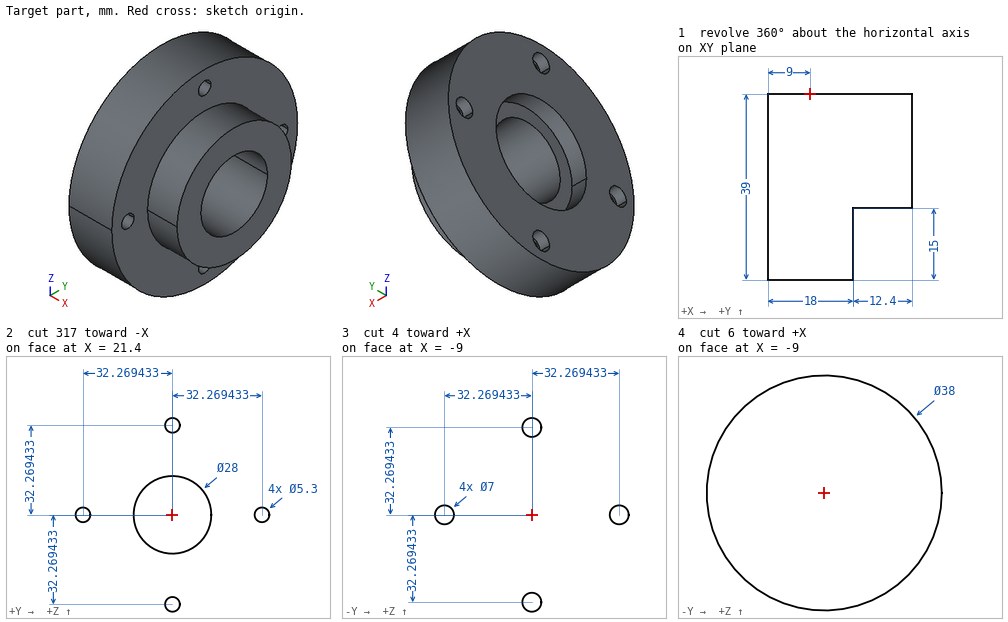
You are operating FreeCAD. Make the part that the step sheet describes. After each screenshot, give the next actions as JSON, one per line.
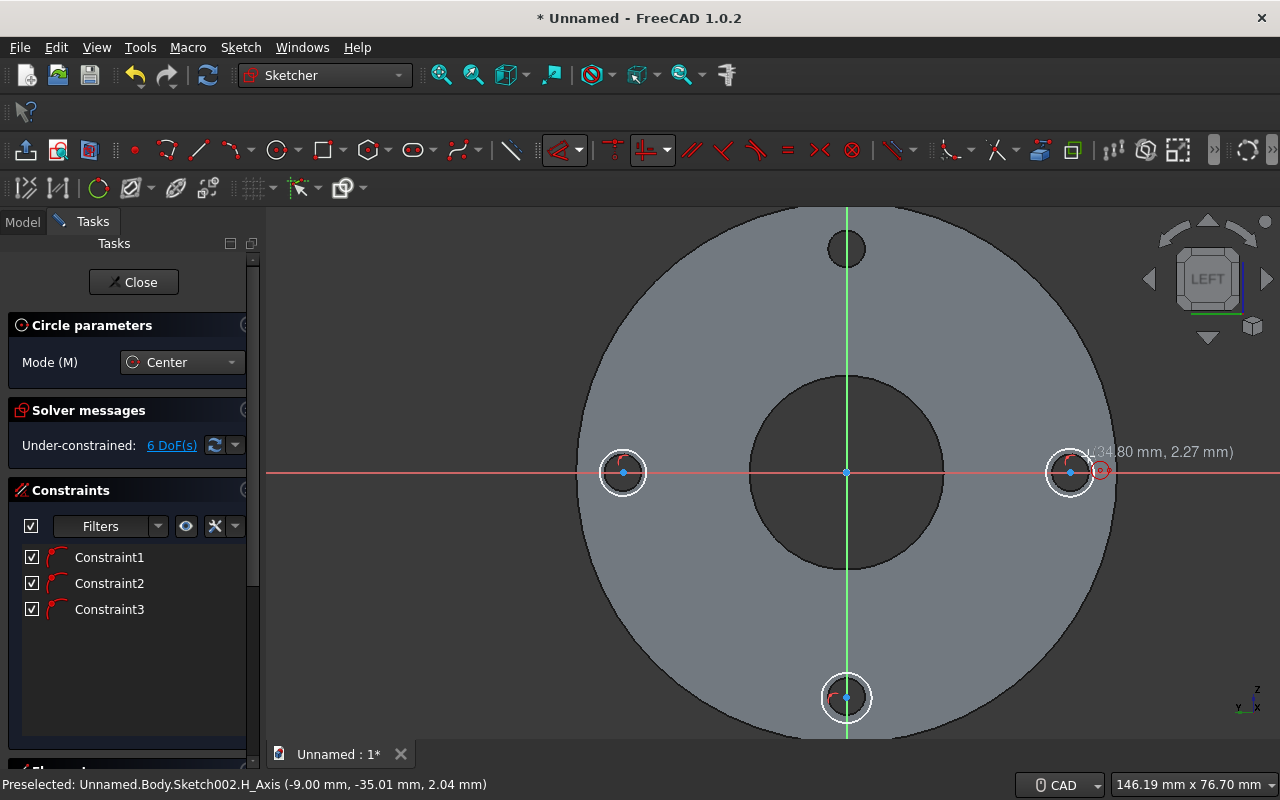
{"action": "left_click", "coordinate": [847, 249]}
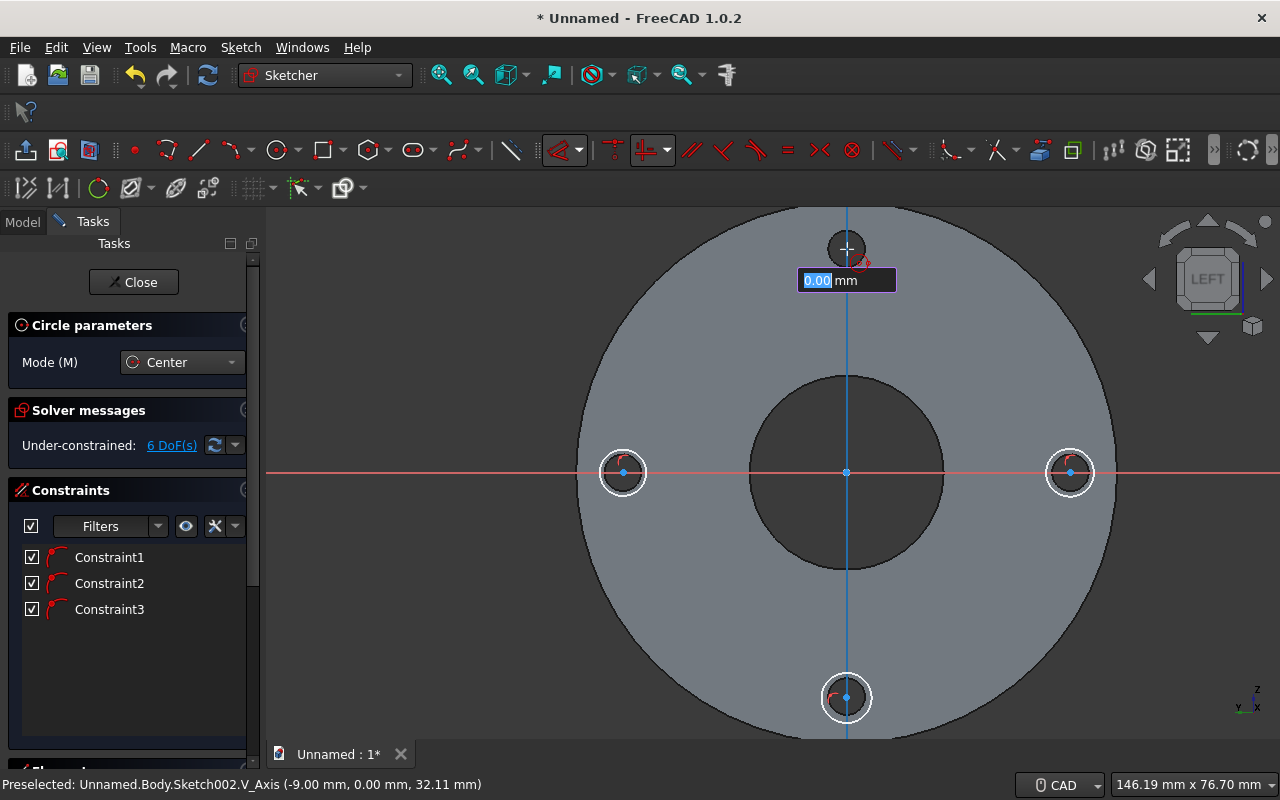
{"action": "scroll", "coordinate": [416, 474], "scroll_direction": "down", "scroll_amount": 2}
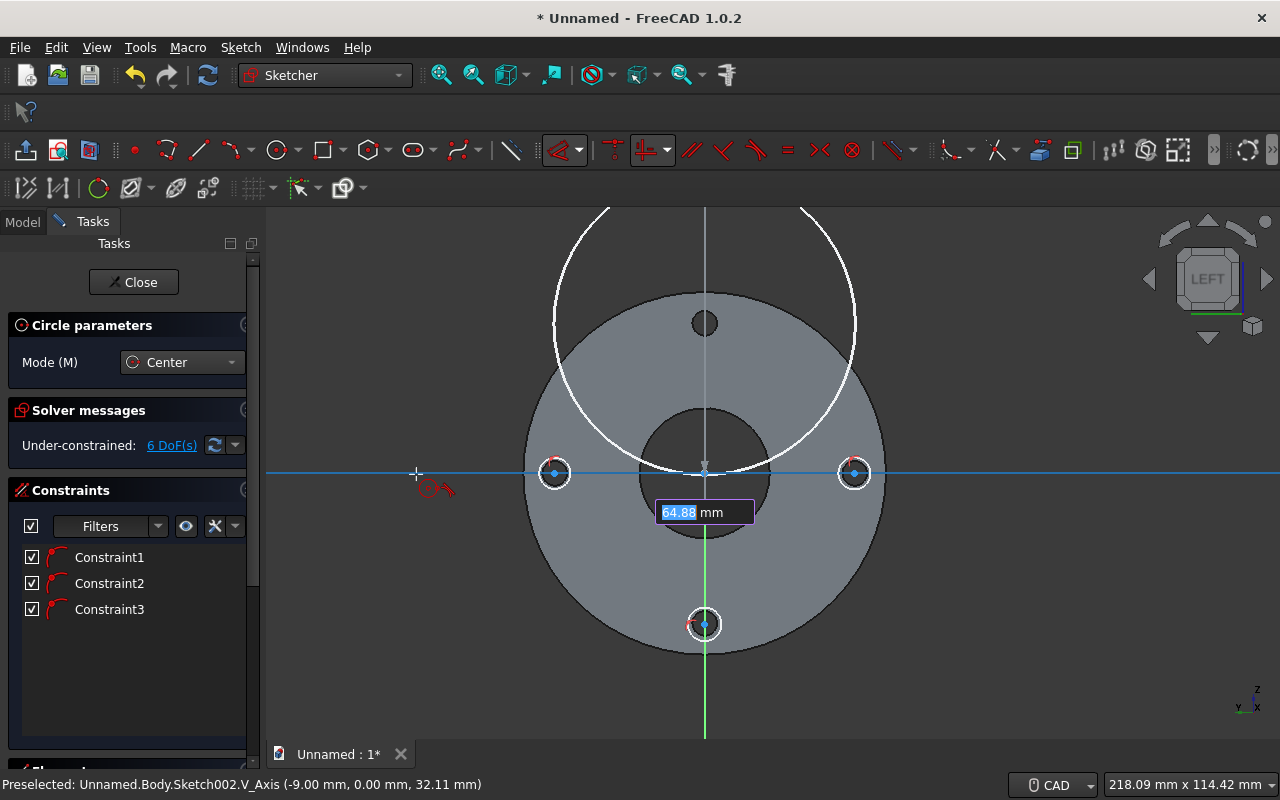
{"action": "scroll", "coordinate": [716, 312], "scroll_direction": "up", "scroll_amount": 2}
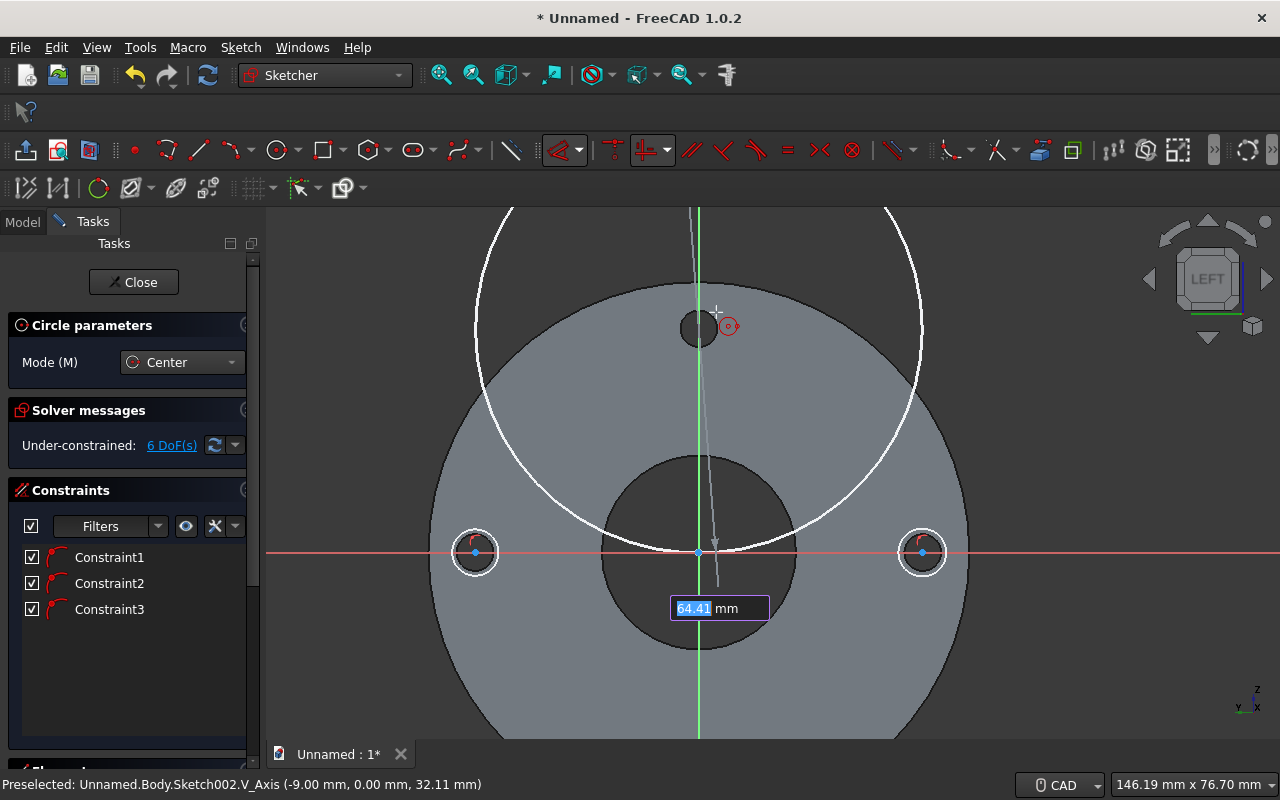
{"action": "left_click", "coordinate": [716, 312]}
{"action": "key", "text": "Escape"}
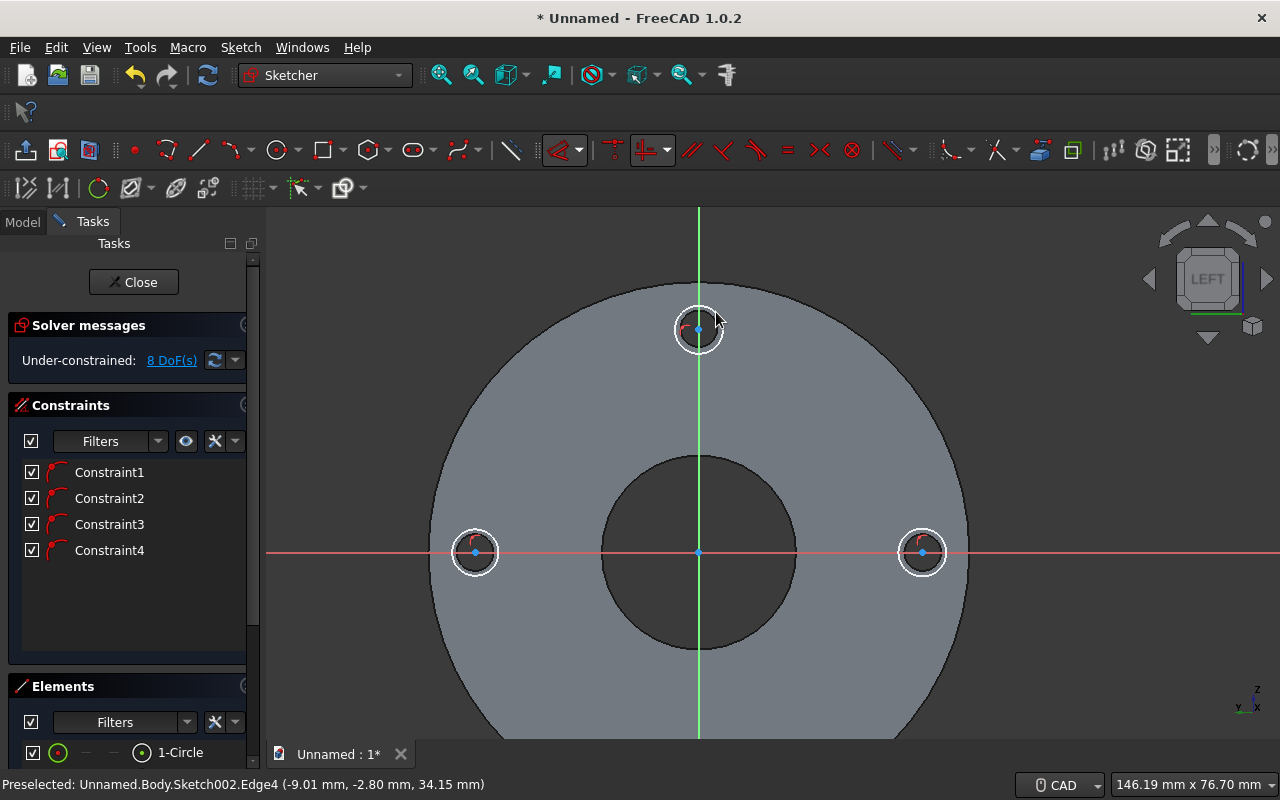
{"action": "left_click", "coordinate": [492, 536]}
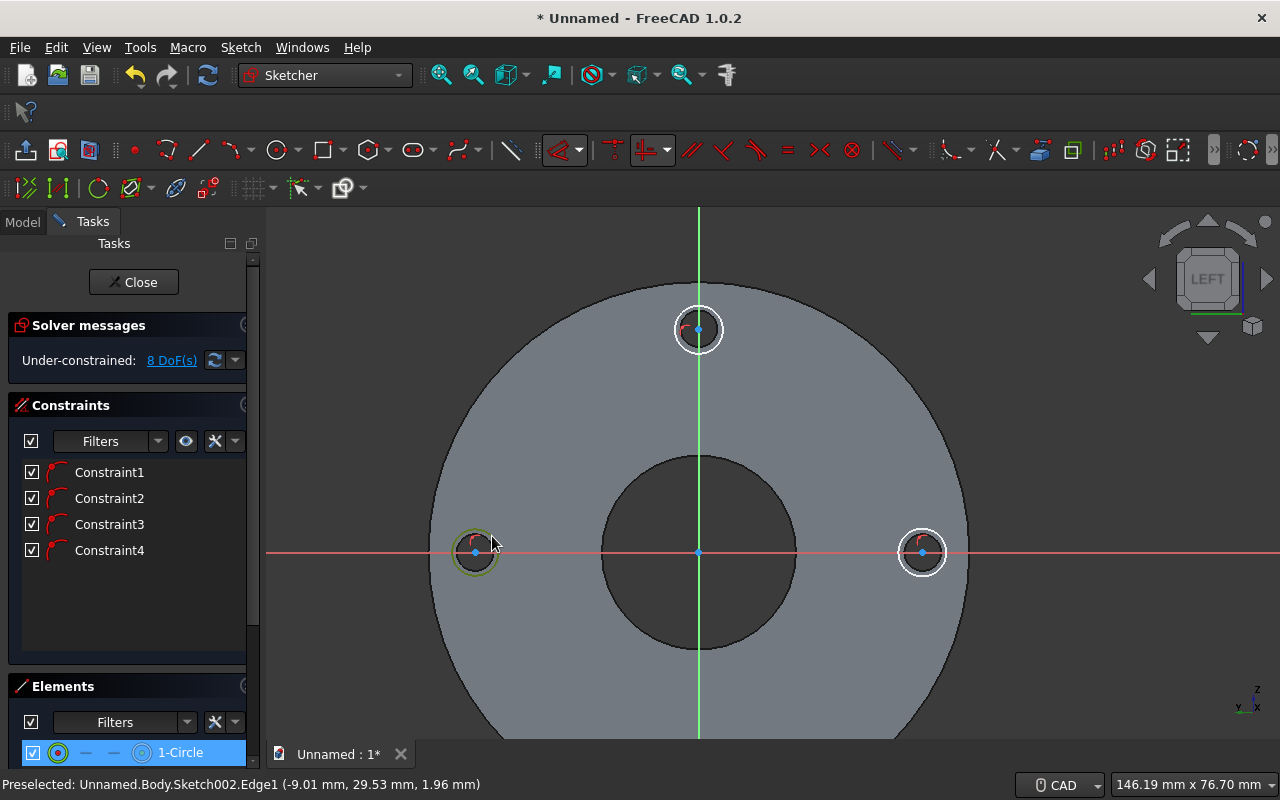
{"action": "scroll", "coordinate": [716, 311], "scroll_direction": "down", "scroll_amount": 2}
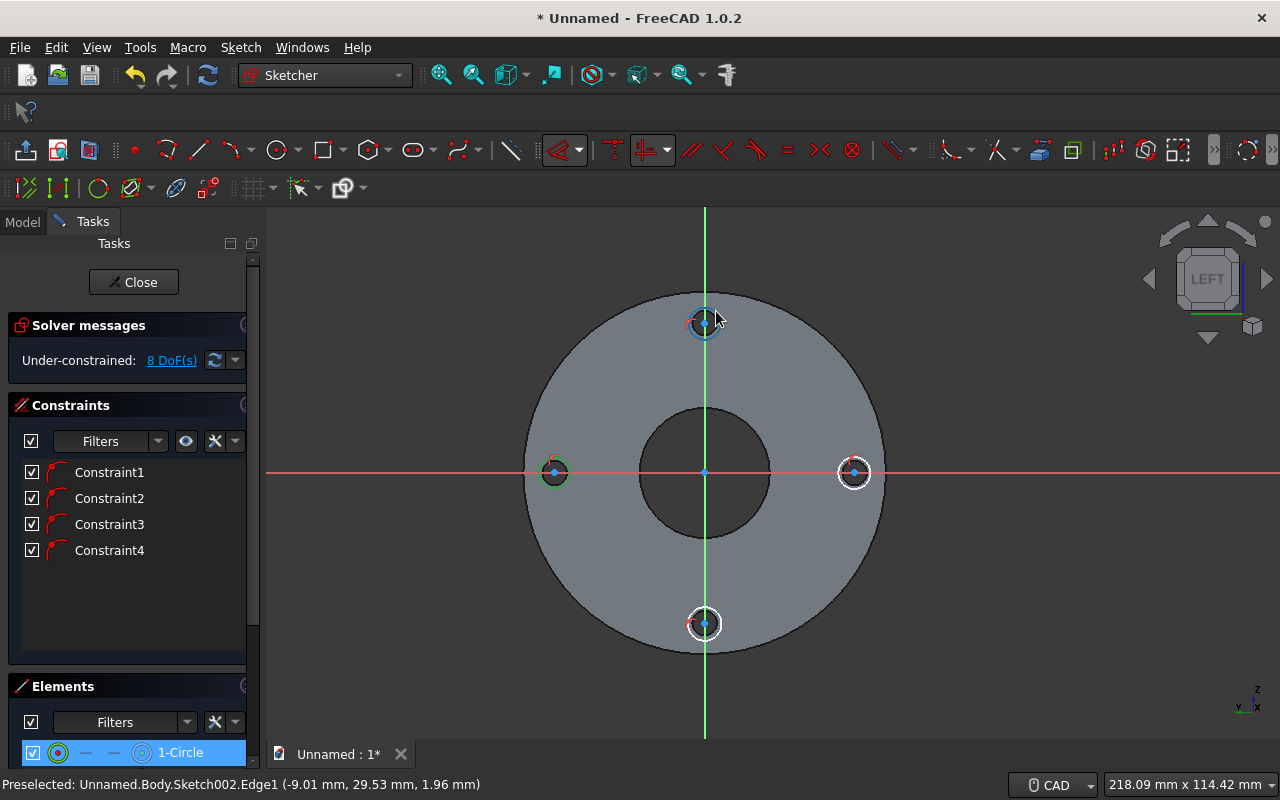
{"action": "left_click", "coordinate": [717, 612]}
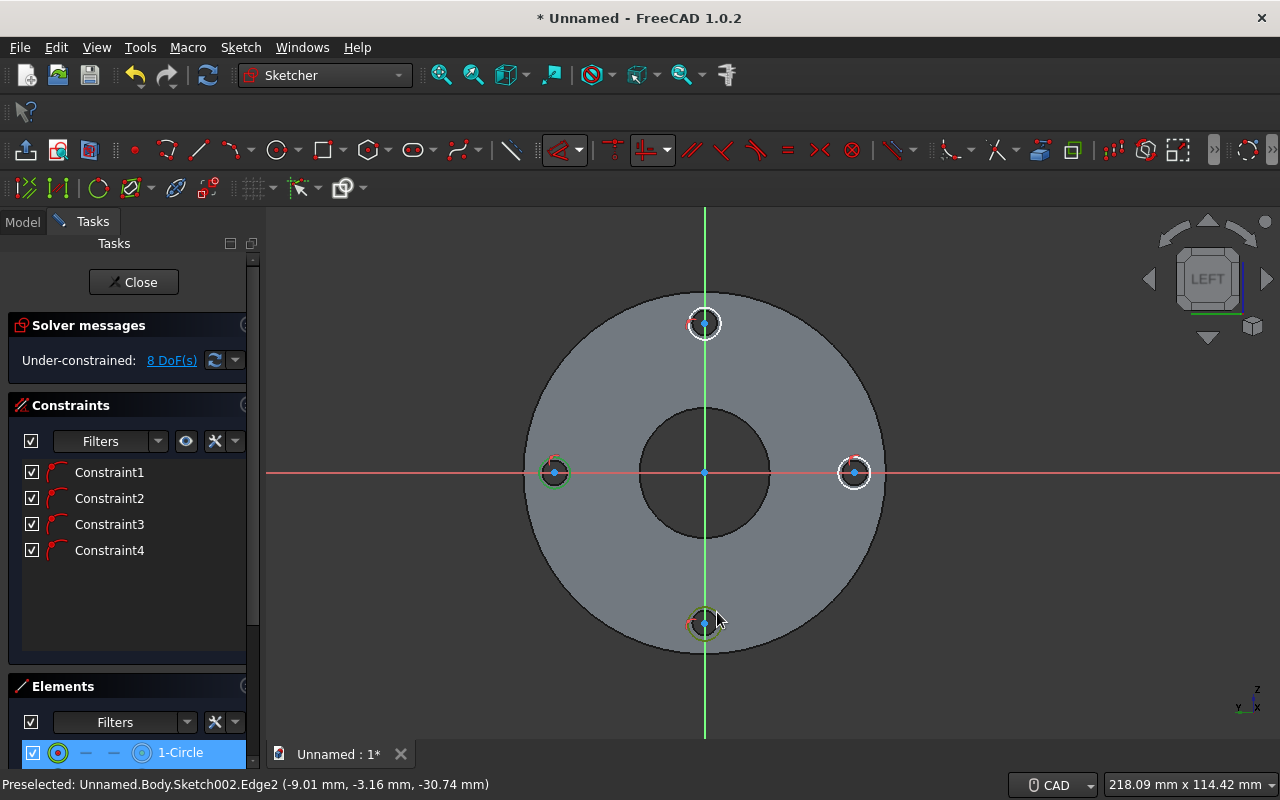
{"action": "left_click", "coordinate": [866, 462]}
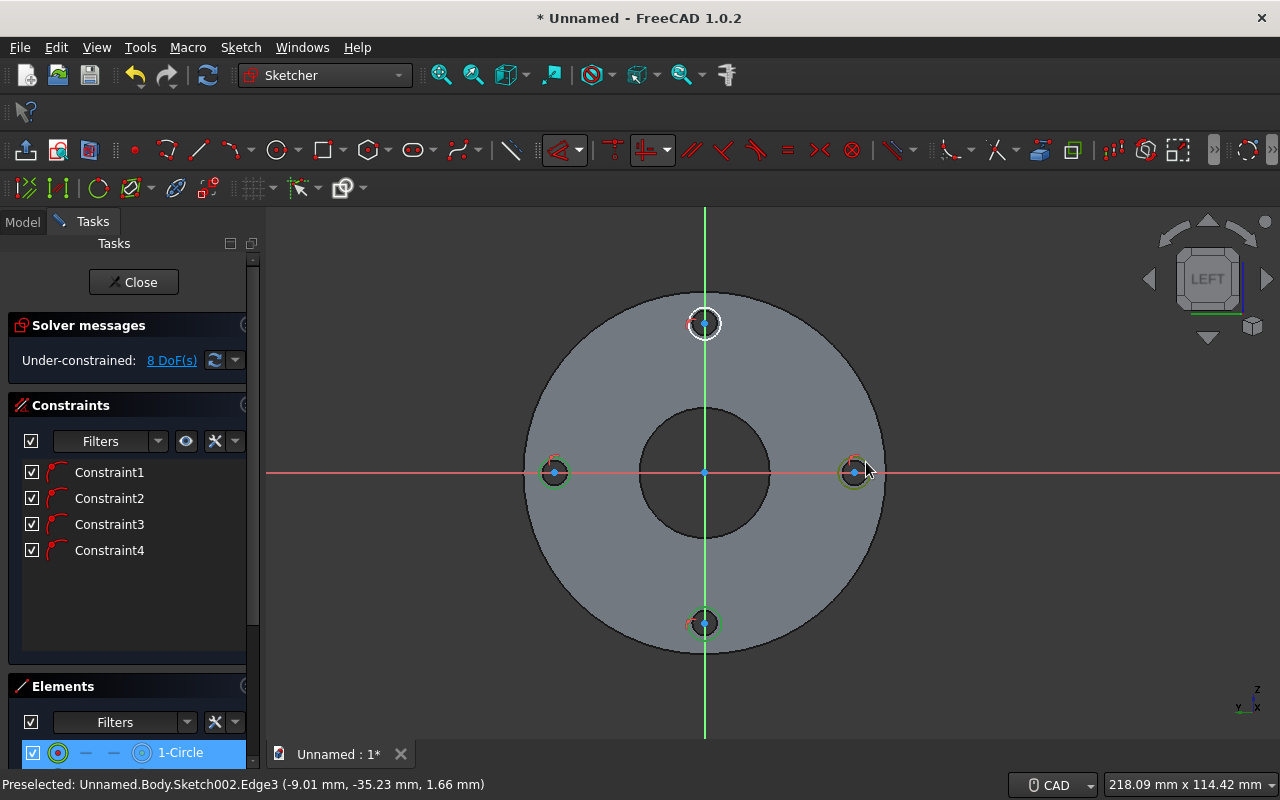
{"action": "left_click", "coordinate": [716, 312]}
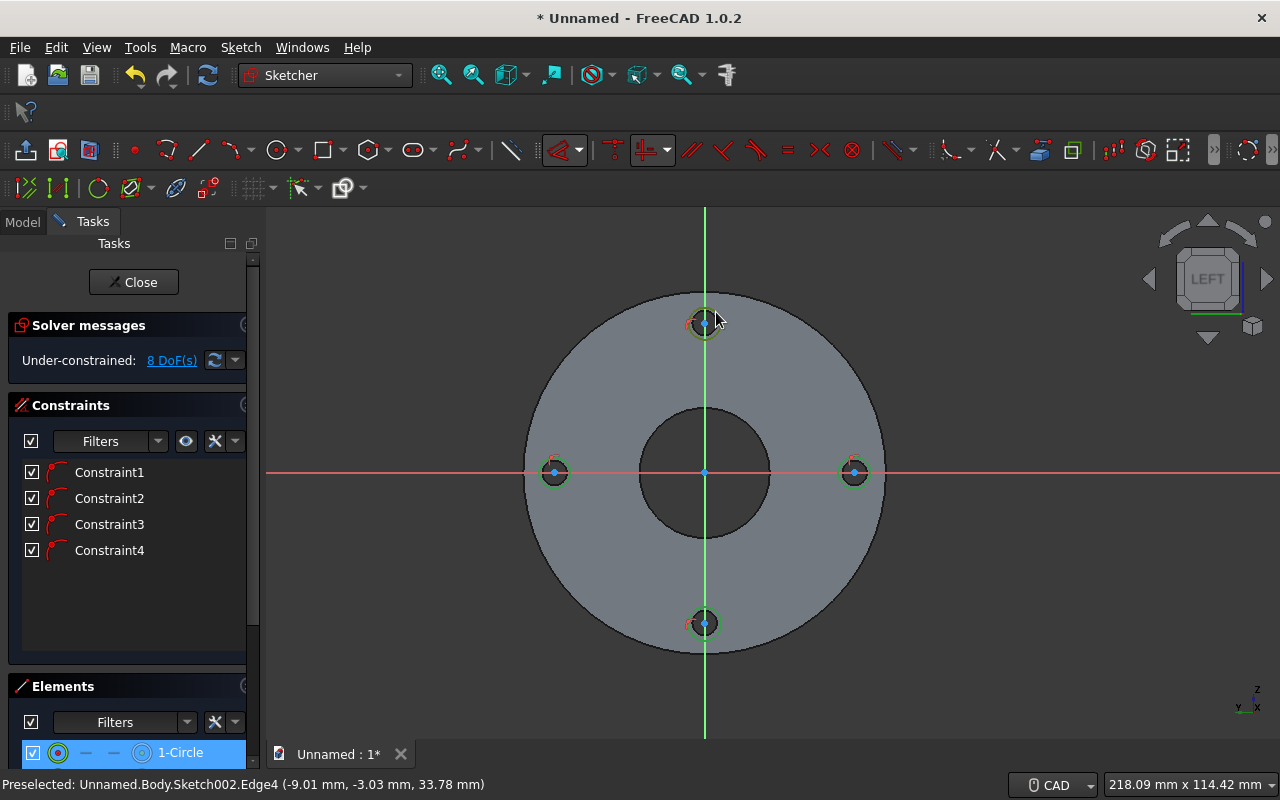
{"action": "left_click", "coordinate": [788, 150]}